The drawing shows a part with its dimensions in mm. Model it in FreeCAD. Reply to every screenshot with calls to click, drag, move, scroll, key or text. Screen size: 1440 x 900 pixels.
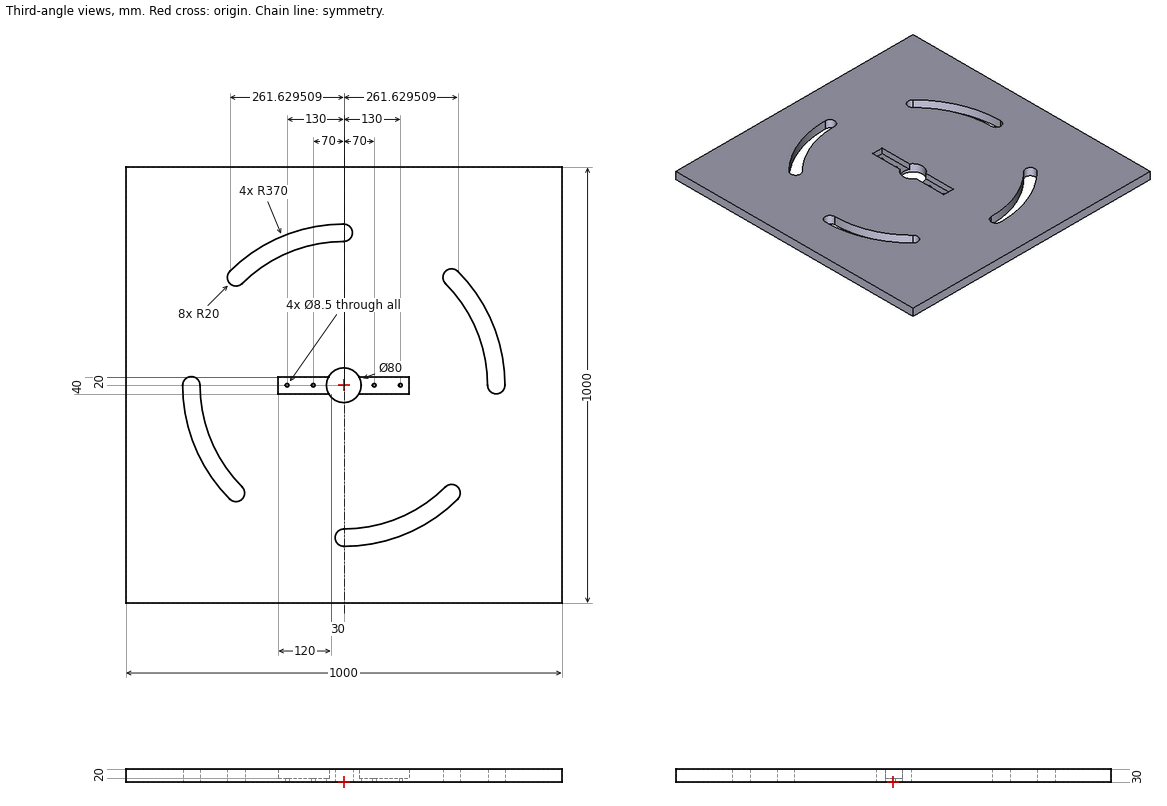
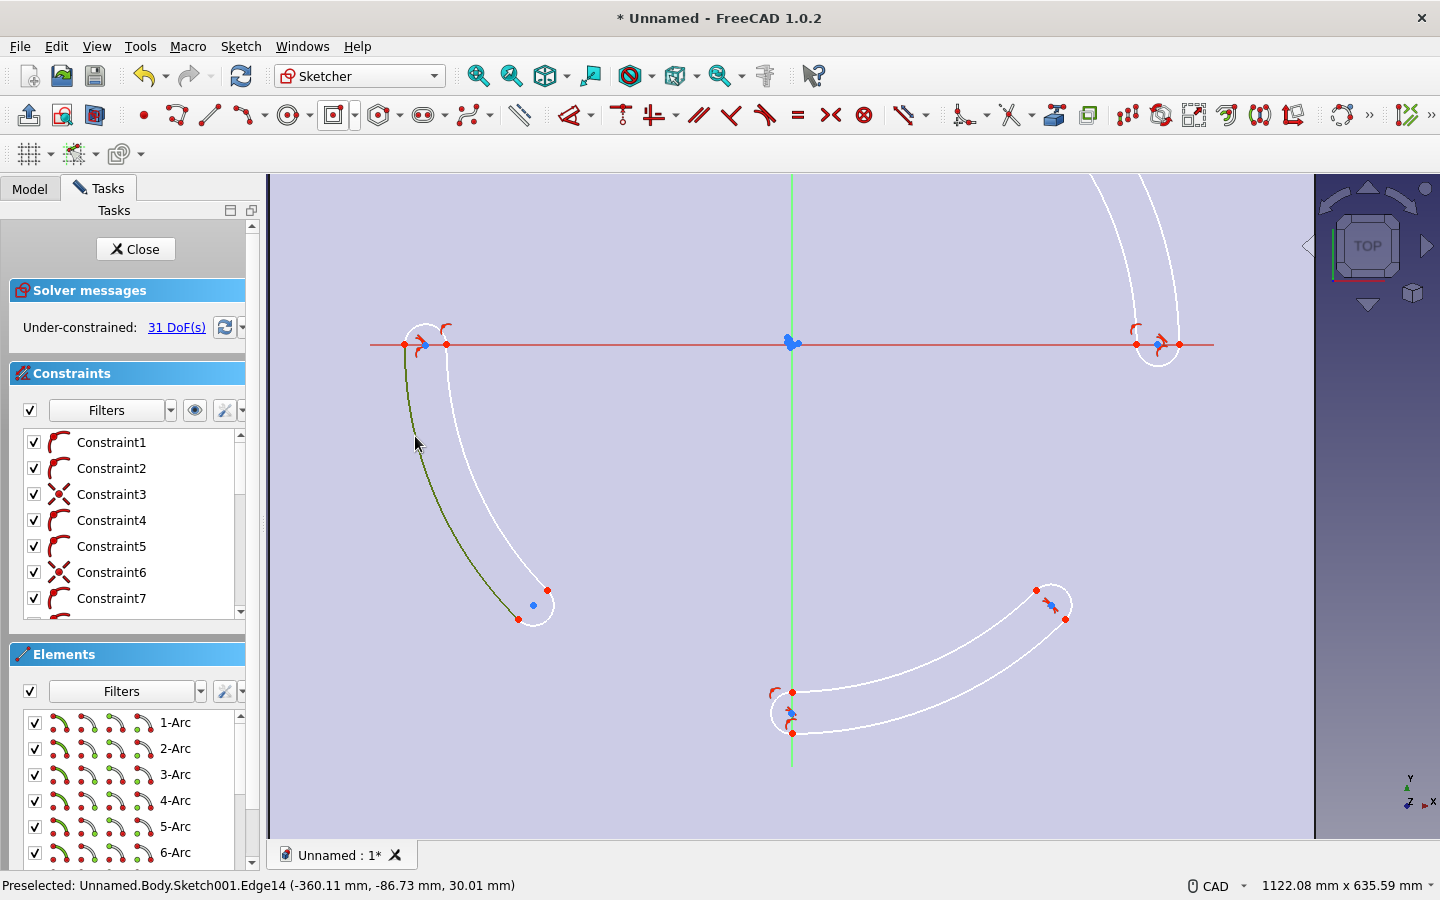
click(536, 626)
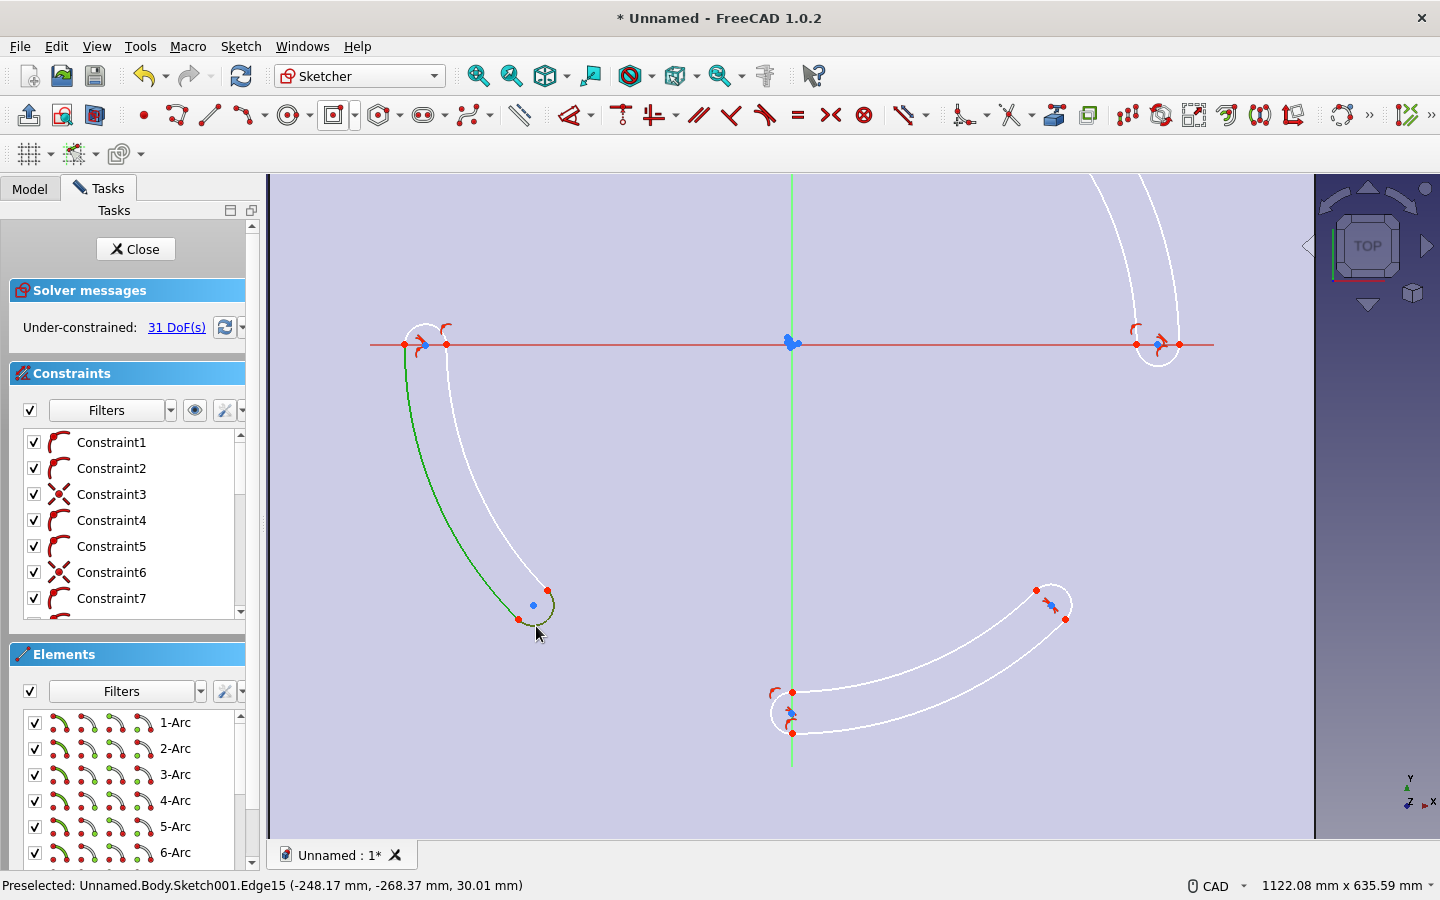
key(t)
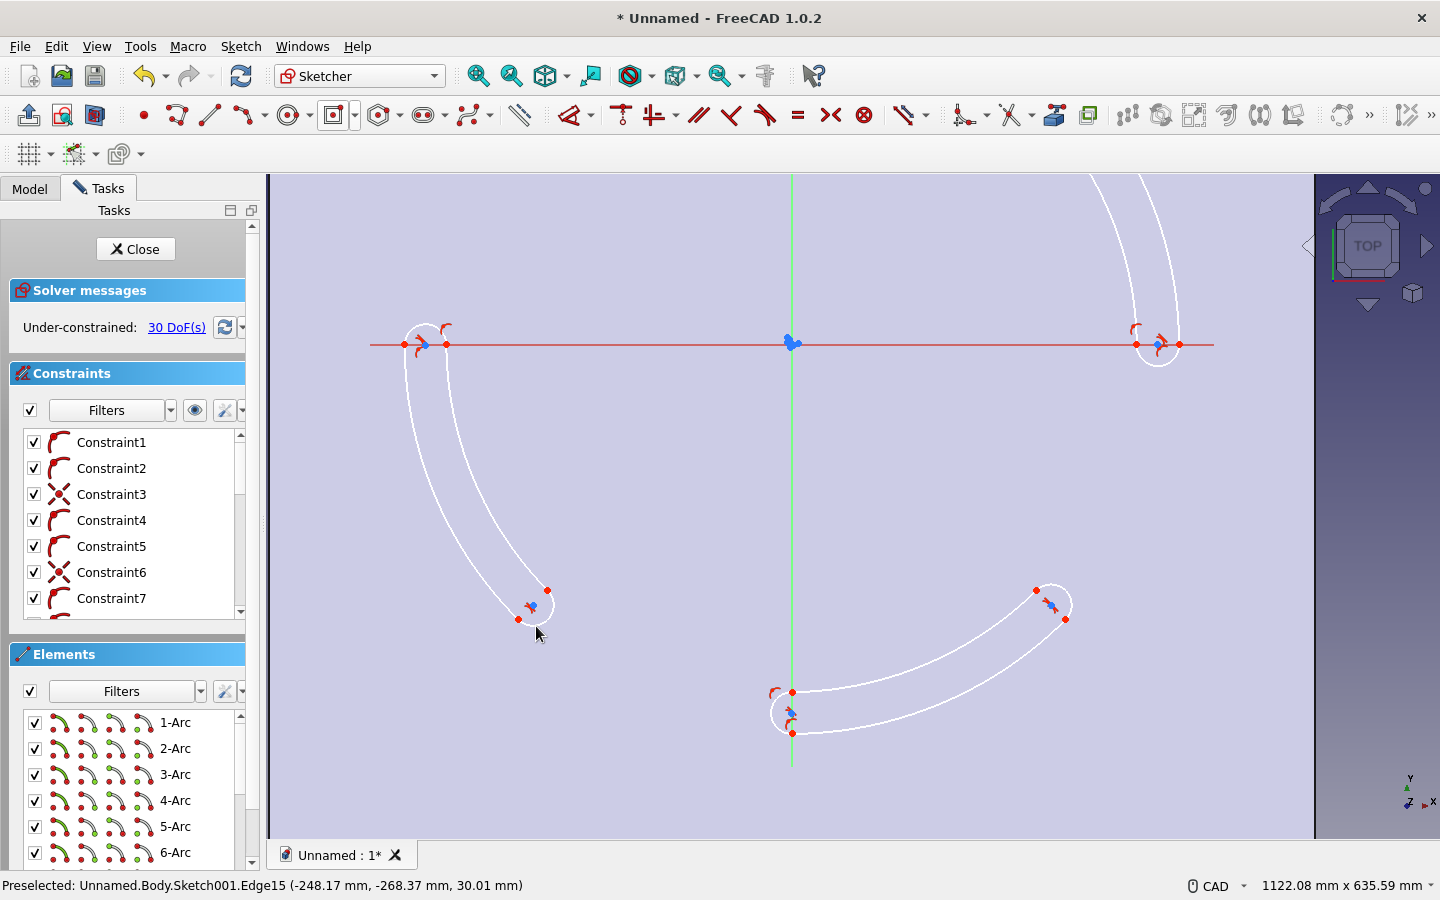
click(536, 625)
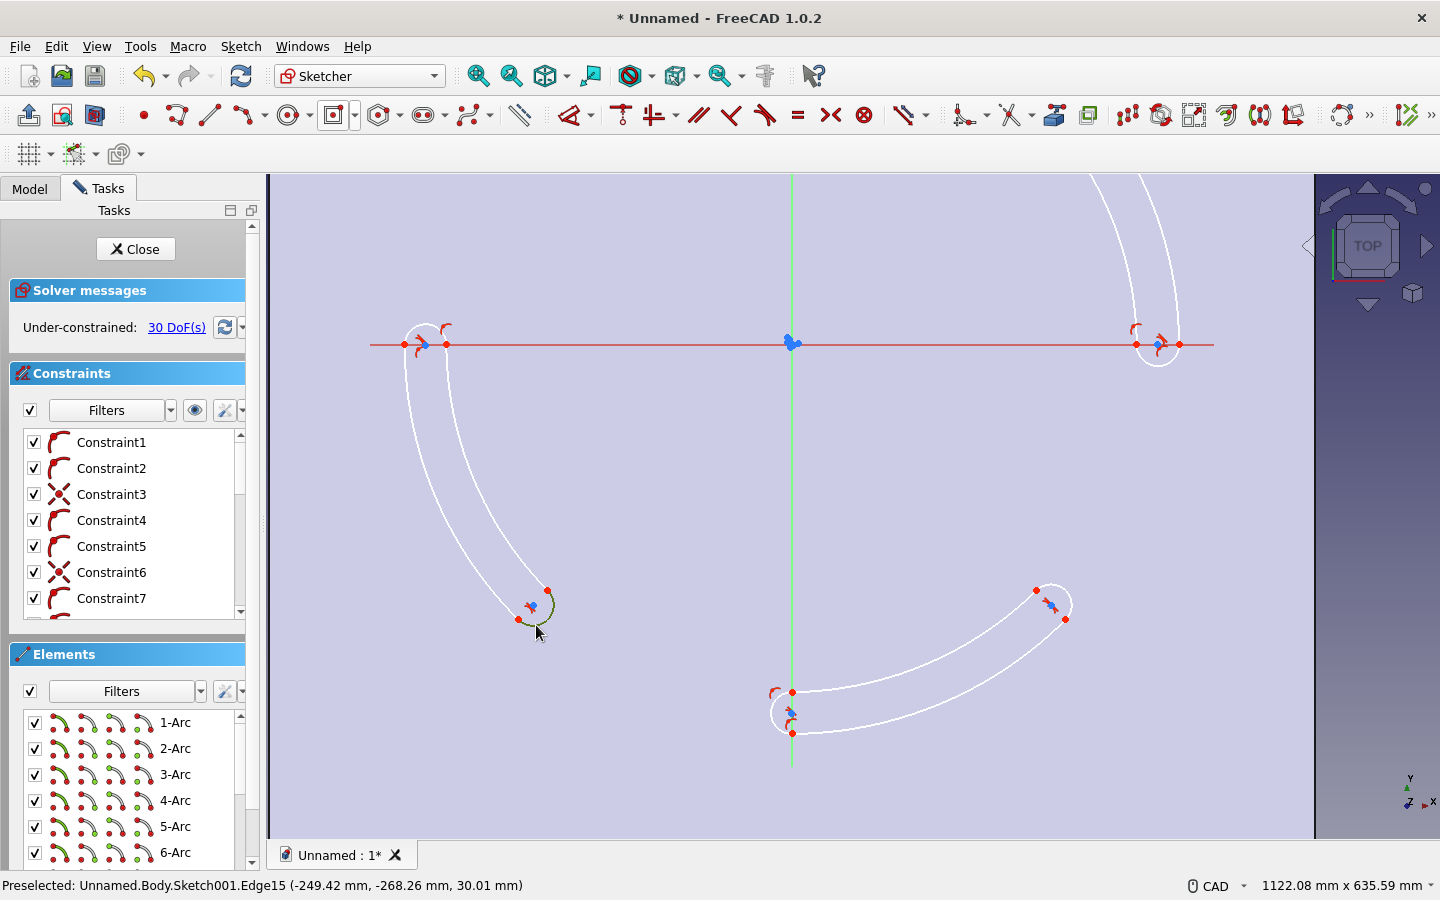
click(456, 426)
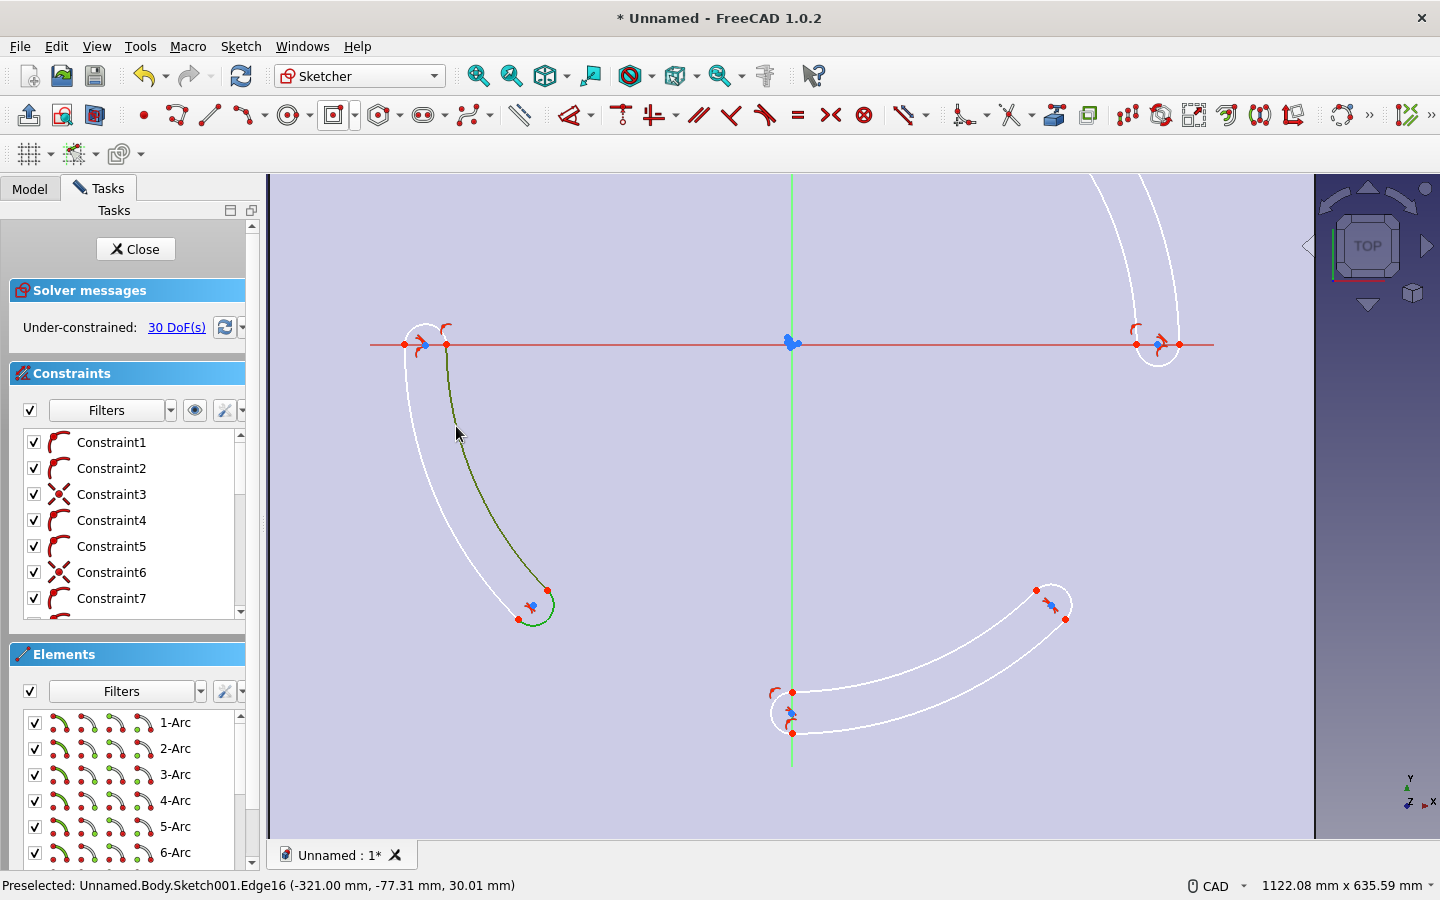
key(t)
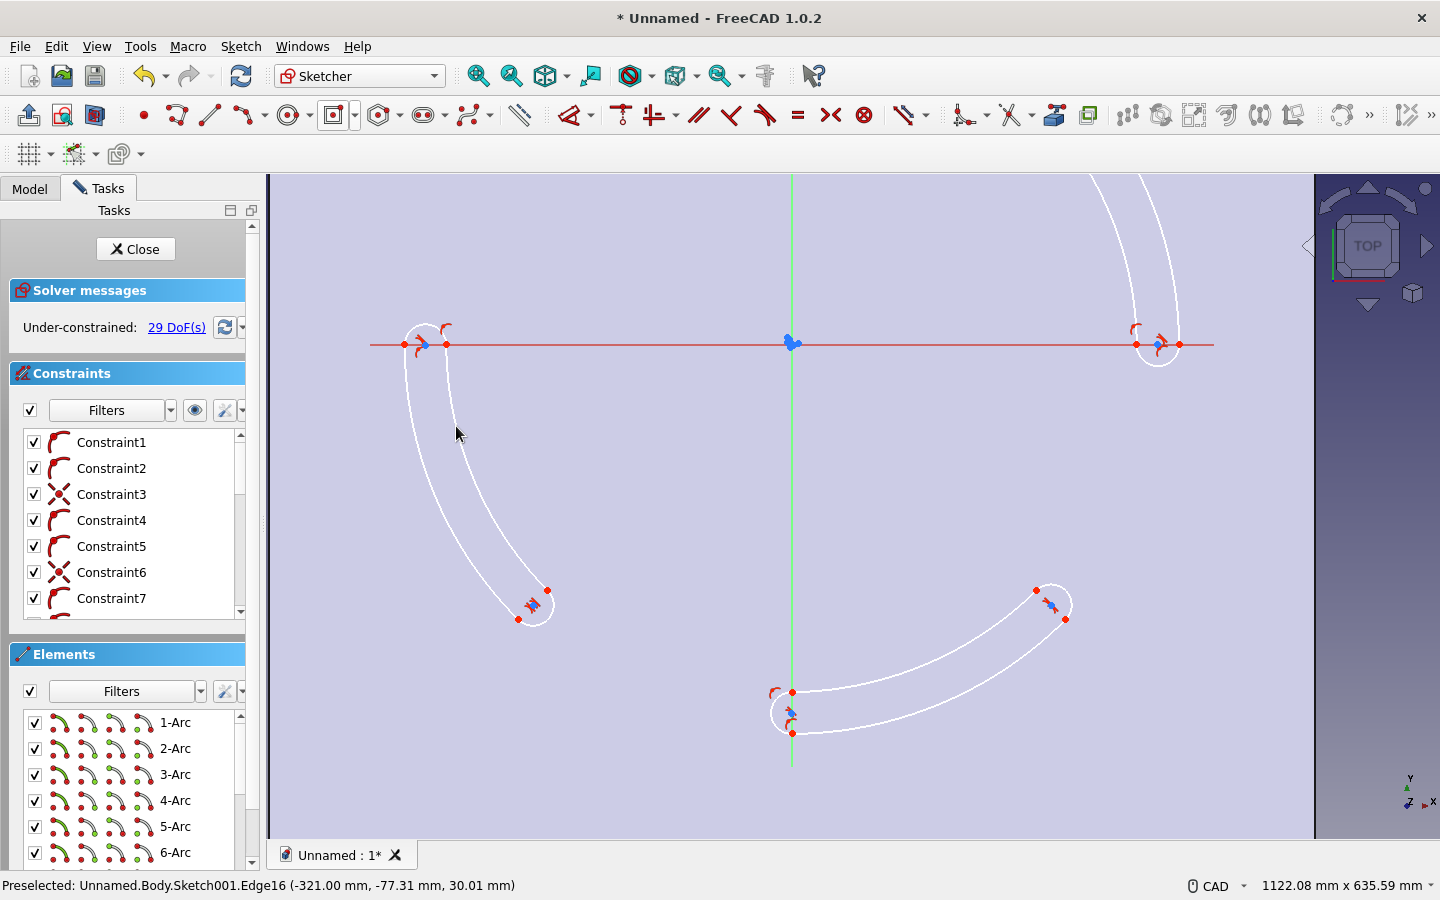
scroll(775, 703, down, 3)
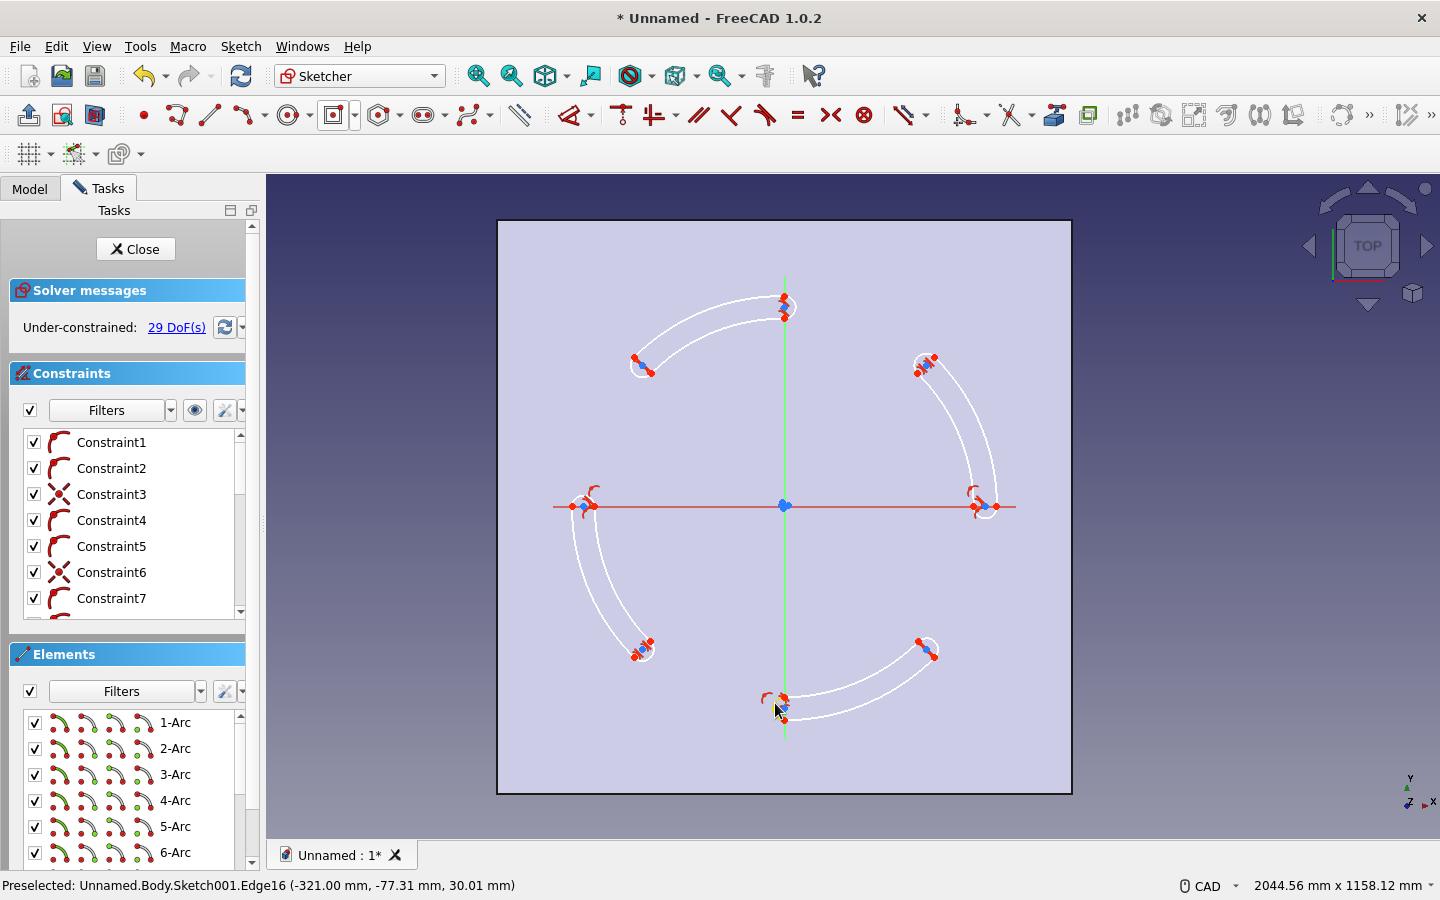
click(735, 301)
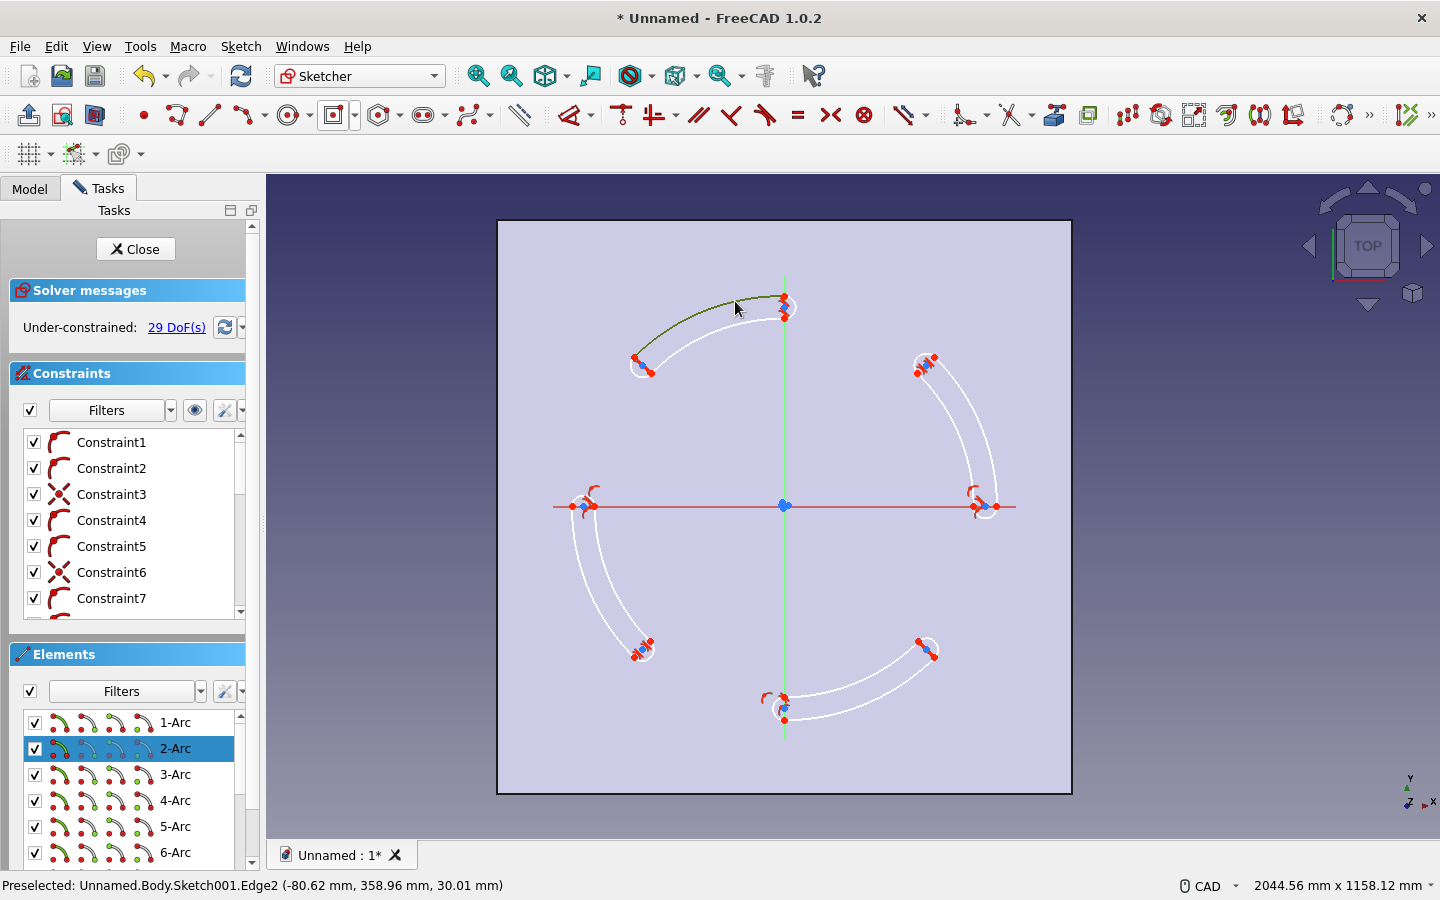
click(740, 324)